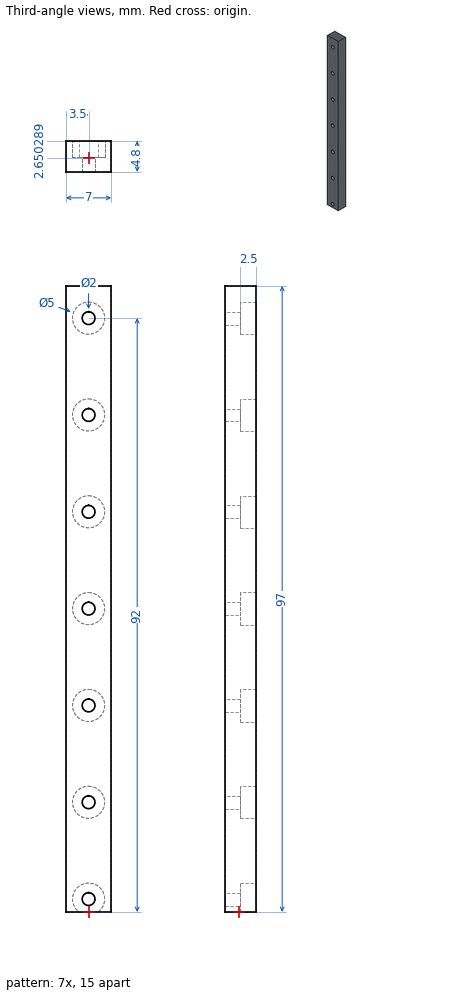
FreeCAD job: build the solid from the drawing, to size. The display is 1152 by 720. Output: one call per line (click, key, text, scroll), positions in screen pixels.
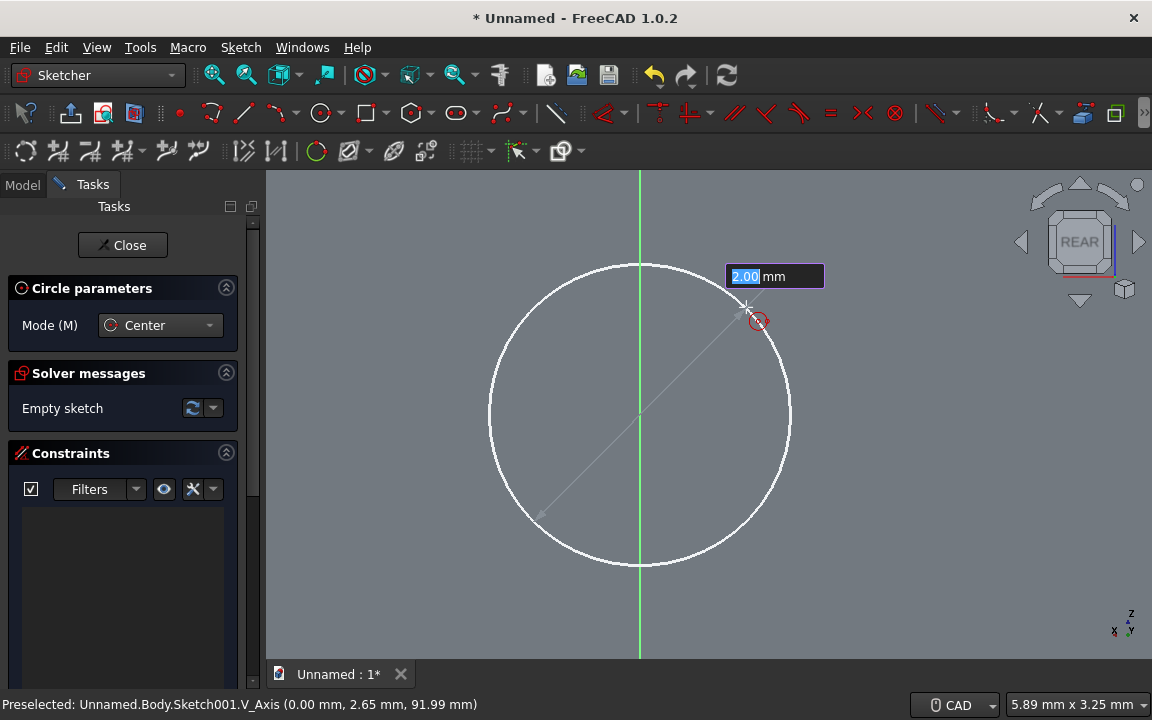
text(2)
key(Return)
key(Escape)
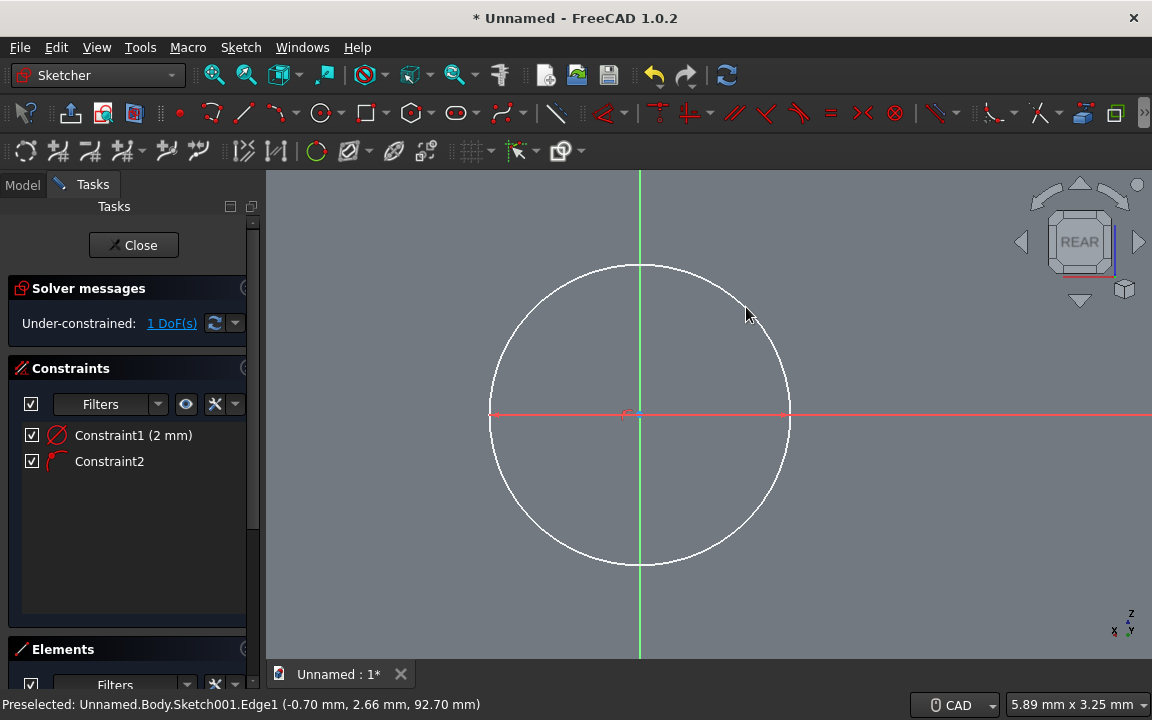
click(604, 114)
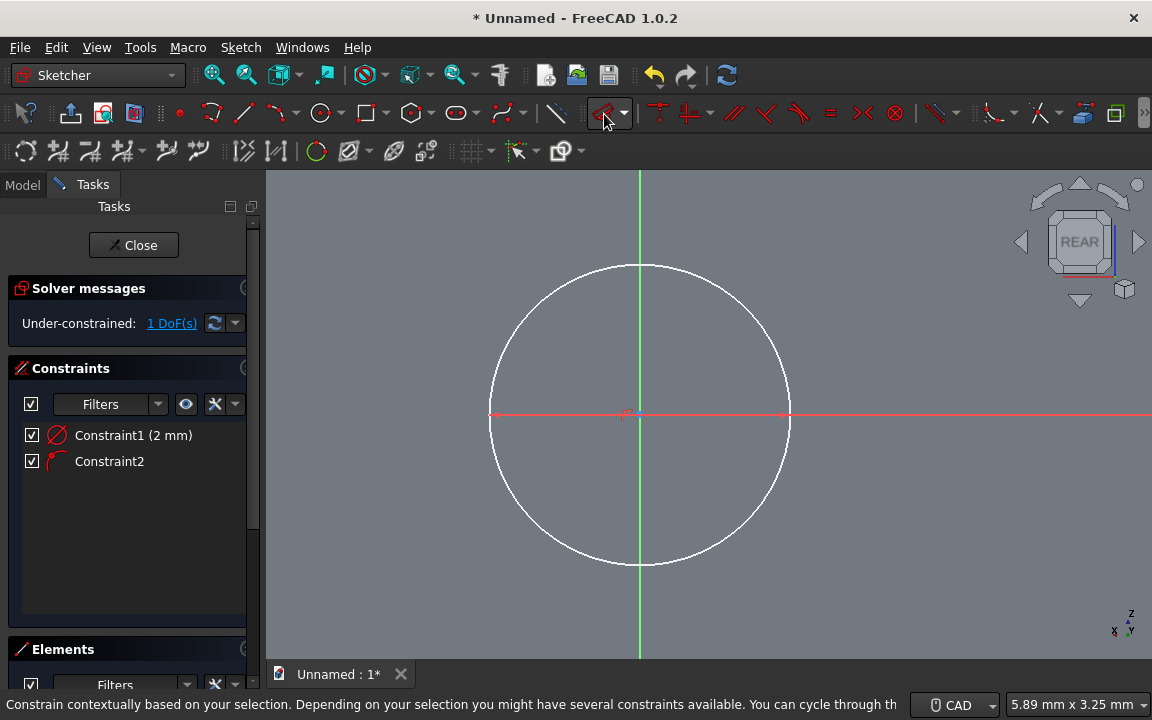
click(640, 415)
click(674, 523)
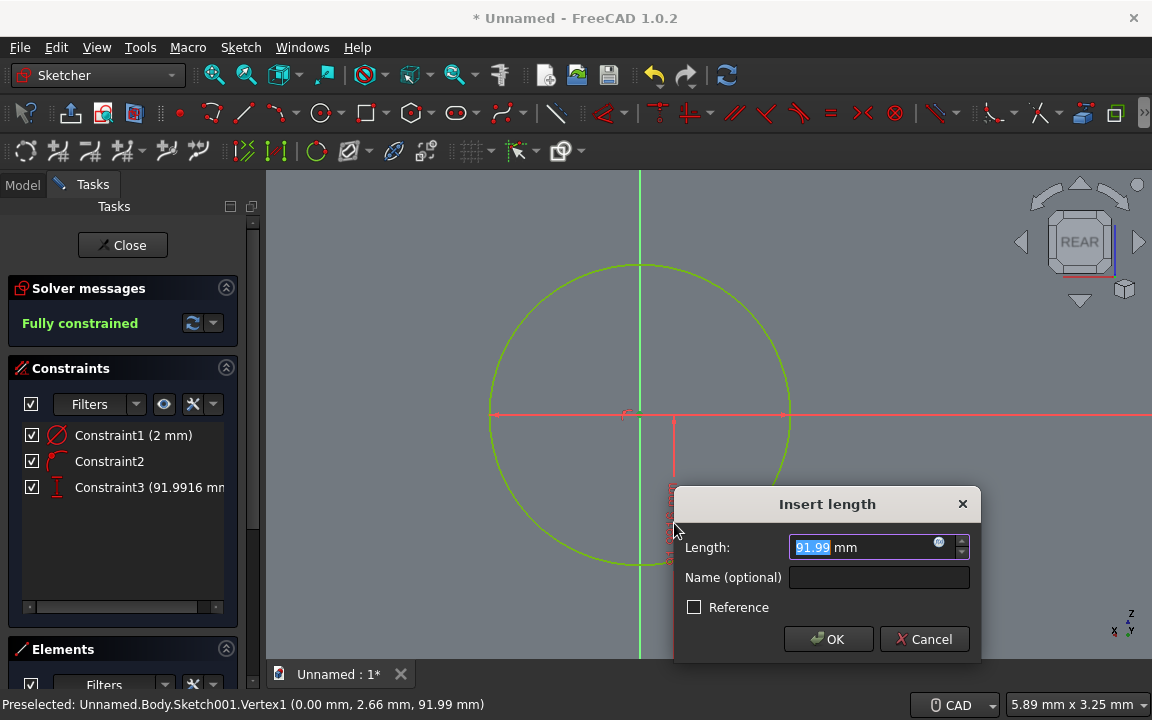
text(92)
key(Return)
key(Escape)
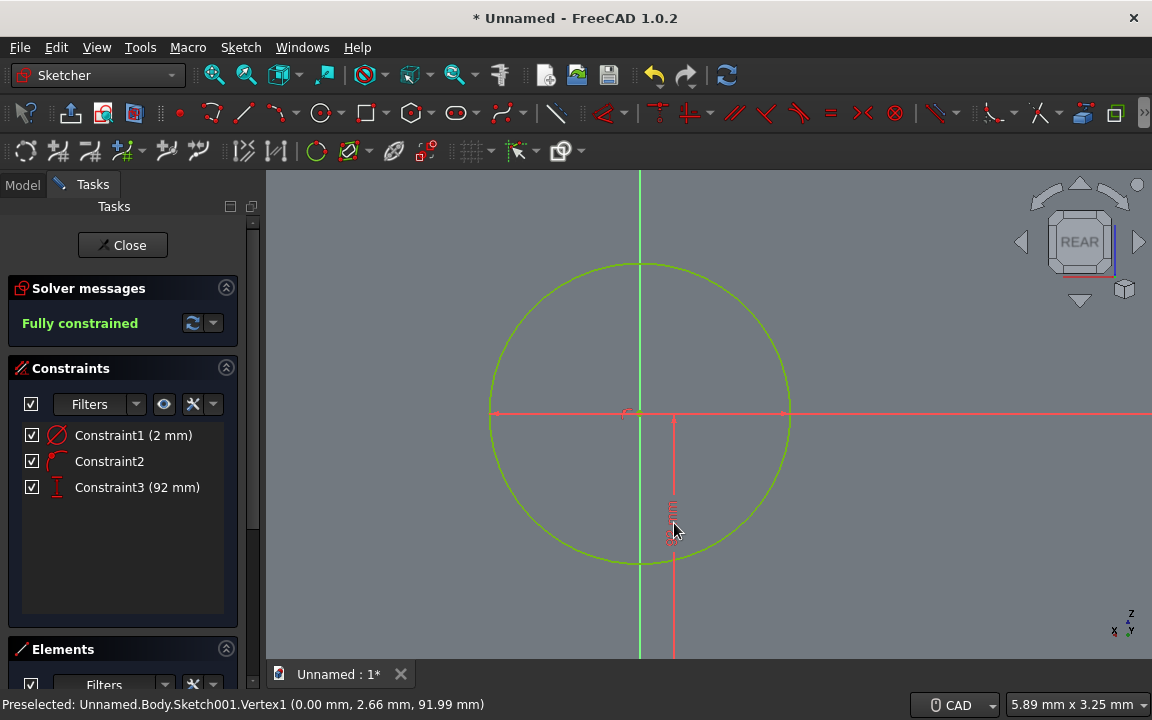
click(123, 245)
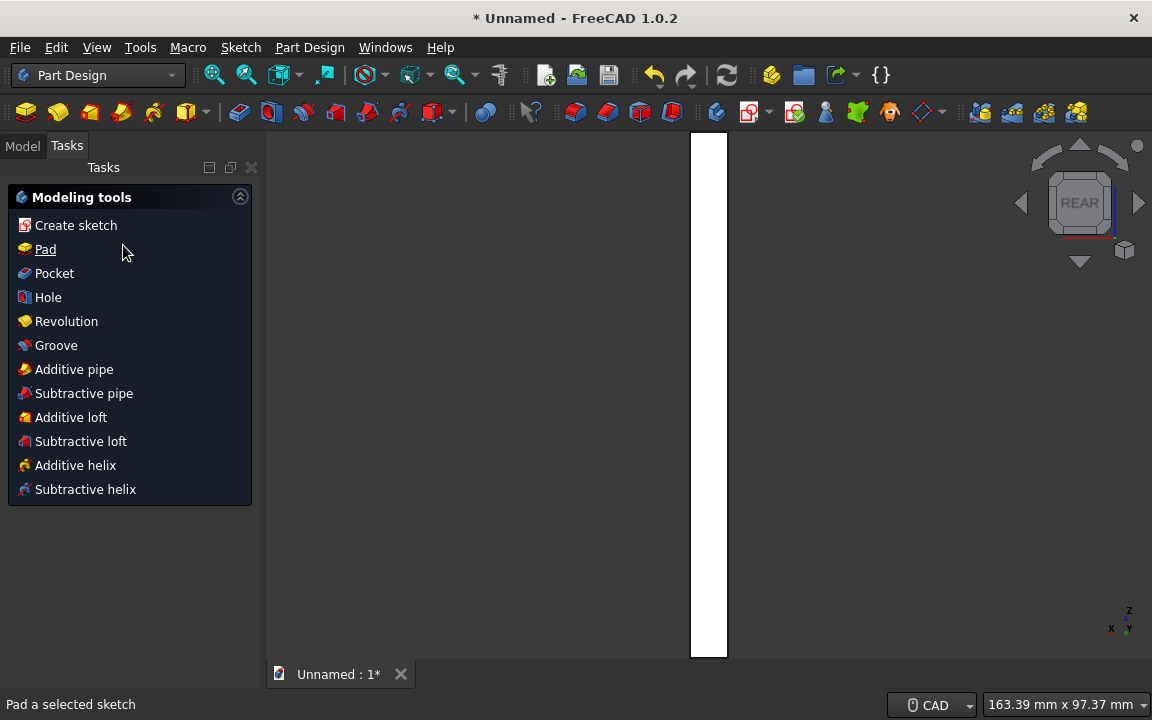
click(240, 112)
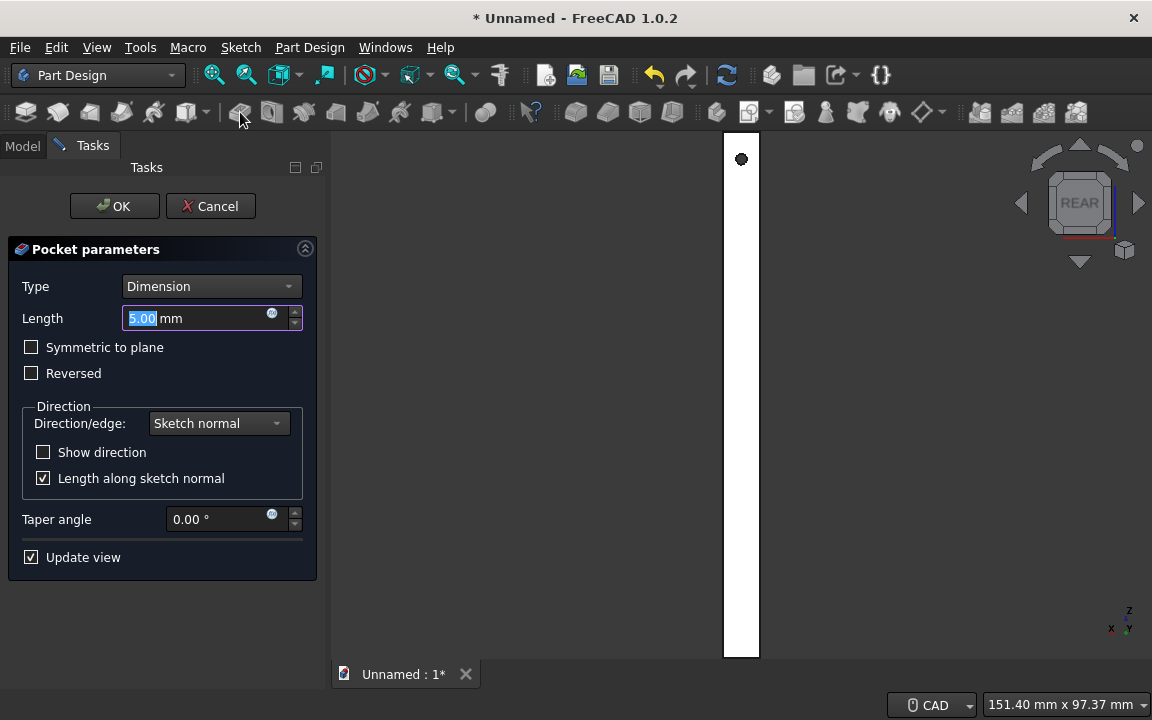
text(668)
key(Tab)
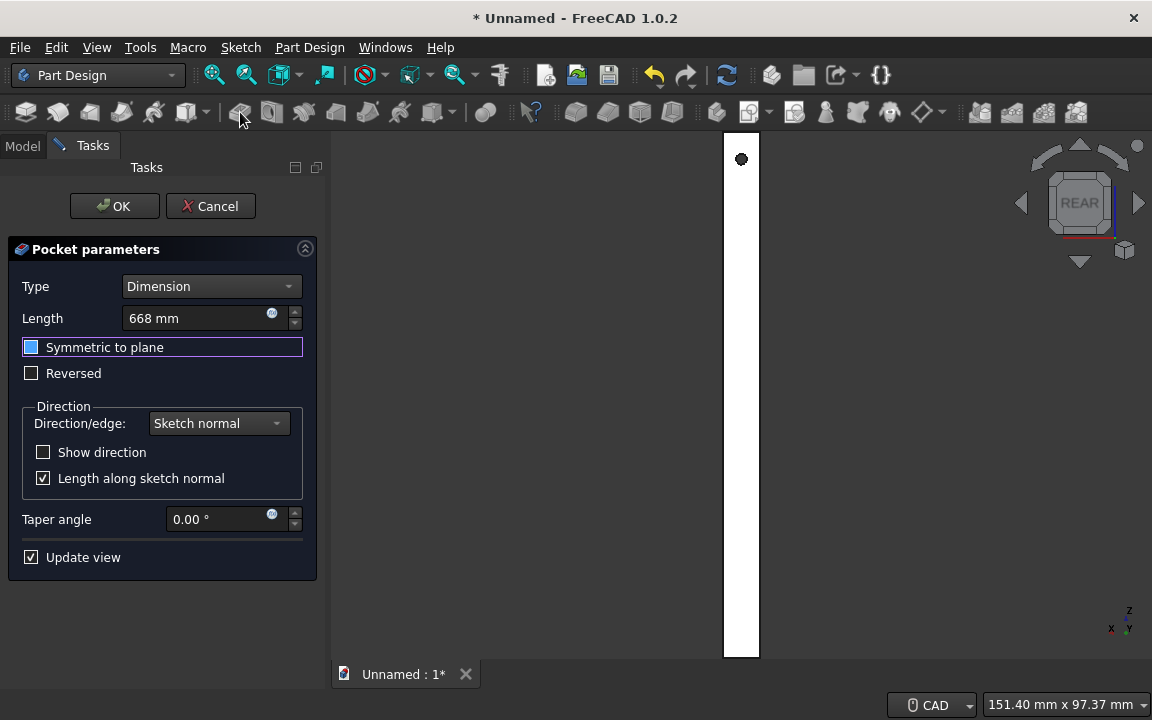
click(115, 206)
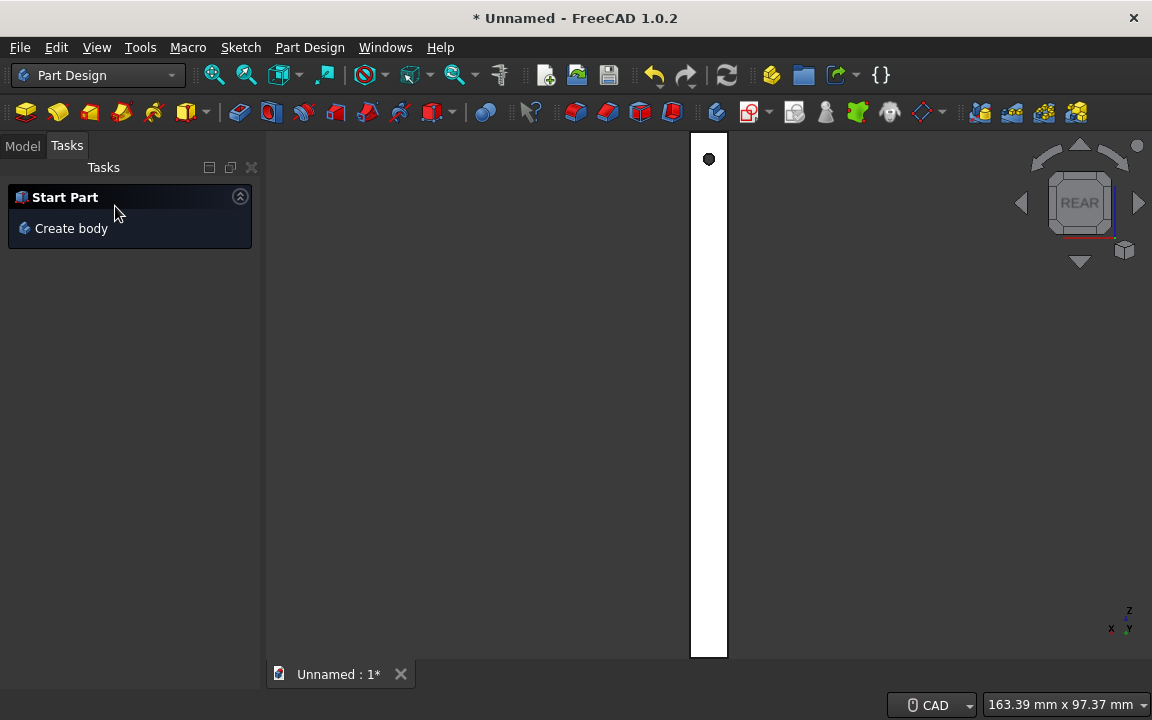
click(709, 244)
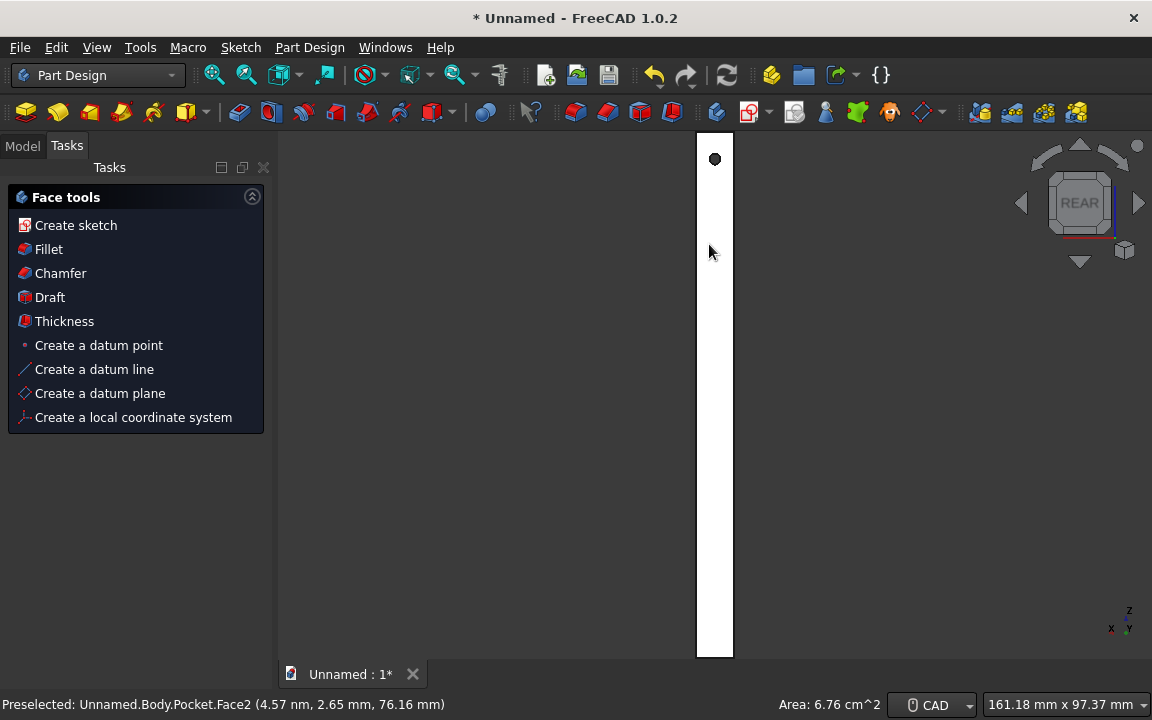
click(750, 112)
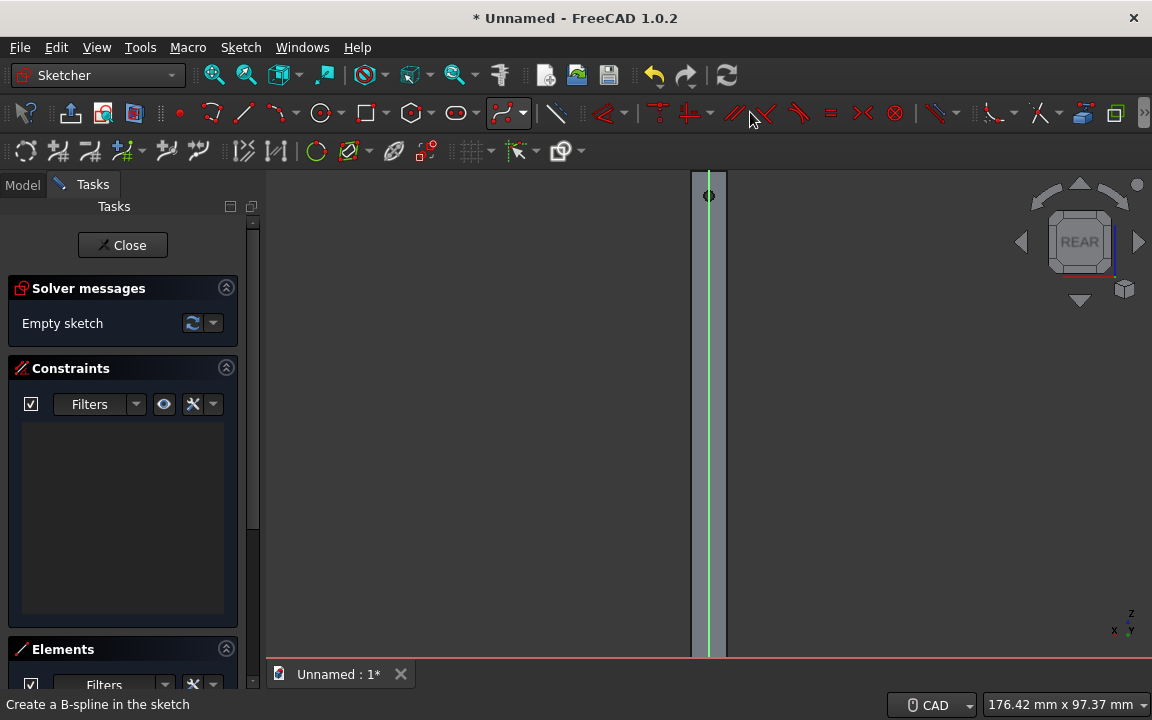
scroll(640, 414, down, 5)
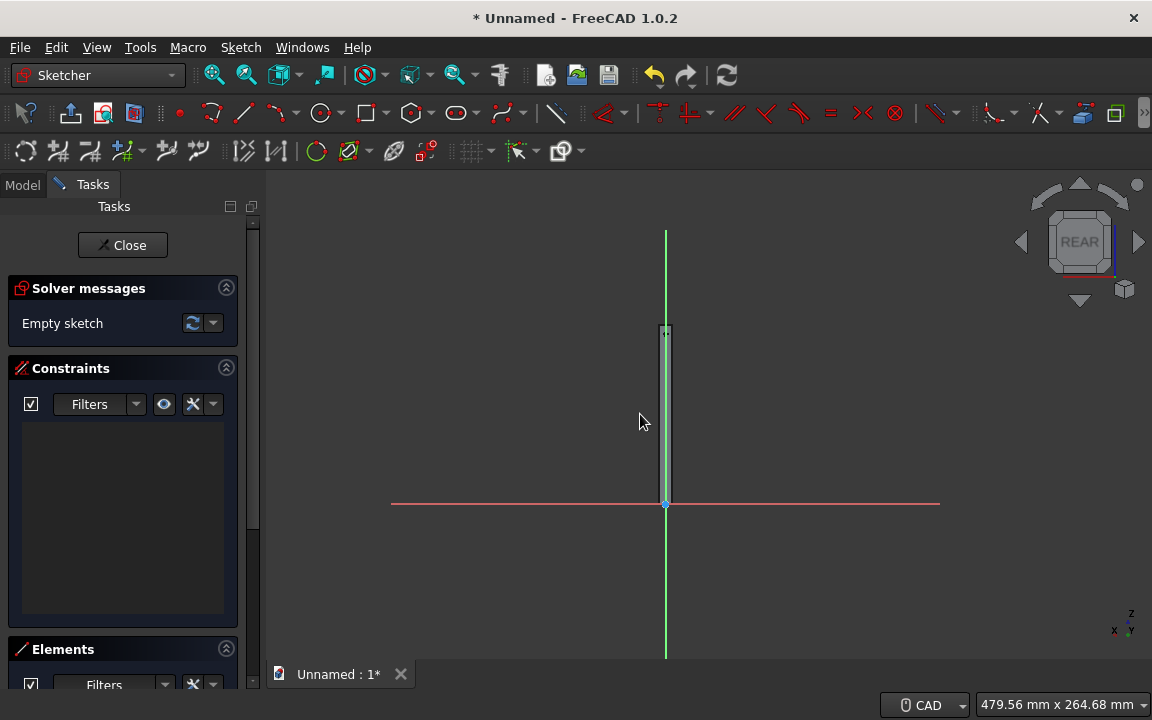
scroll(667, 330, up, 15)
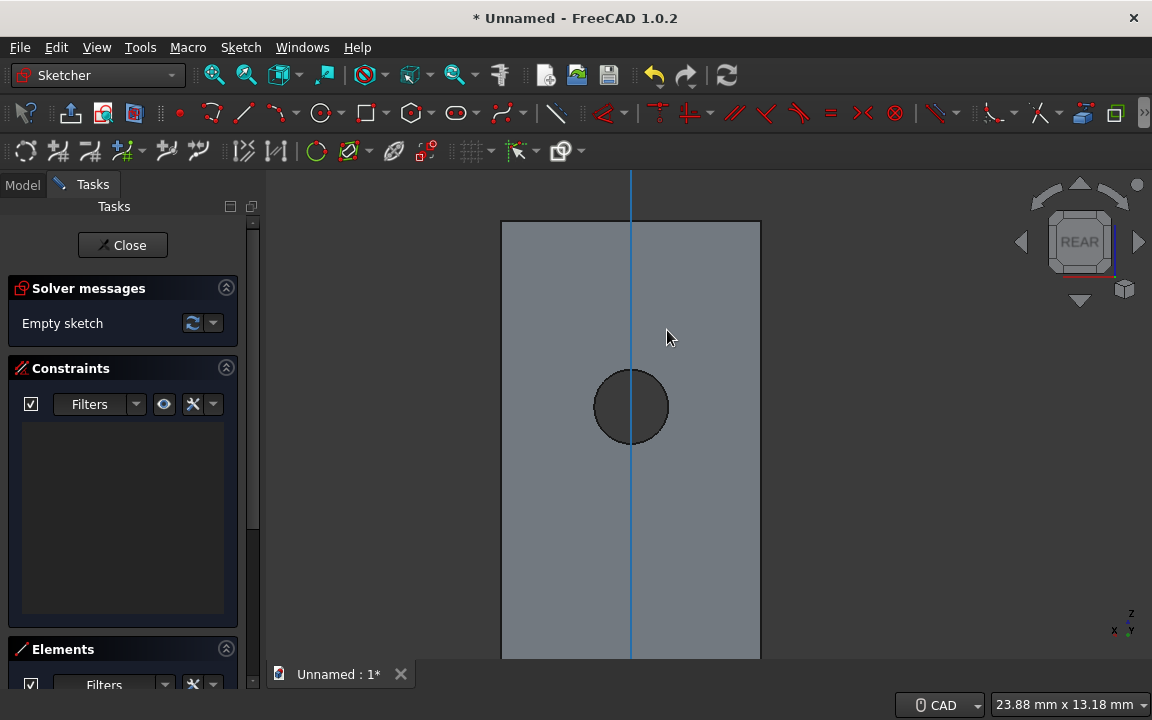
scroll(612, 391, up, 2)